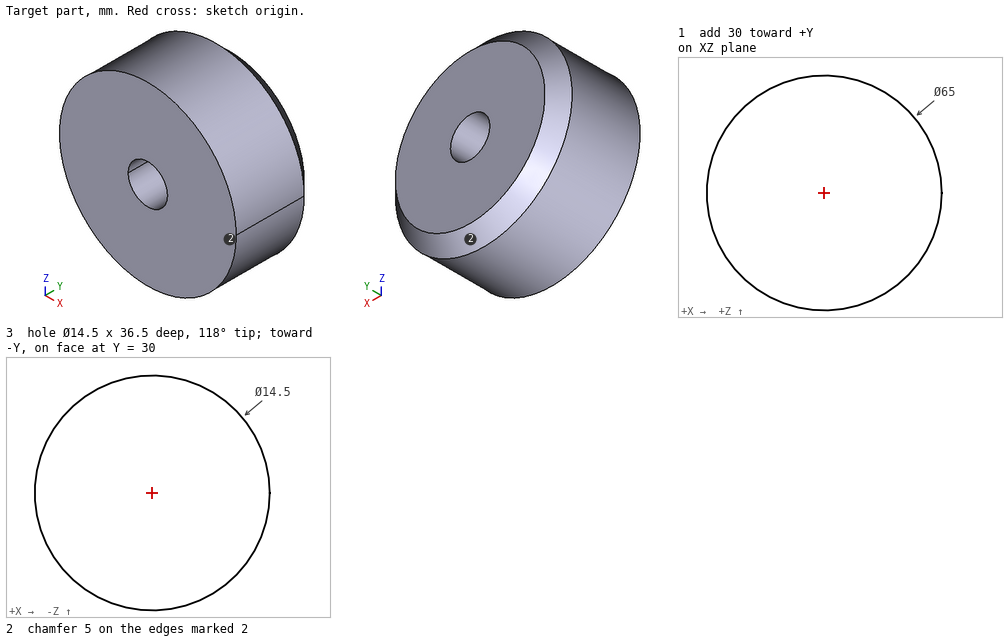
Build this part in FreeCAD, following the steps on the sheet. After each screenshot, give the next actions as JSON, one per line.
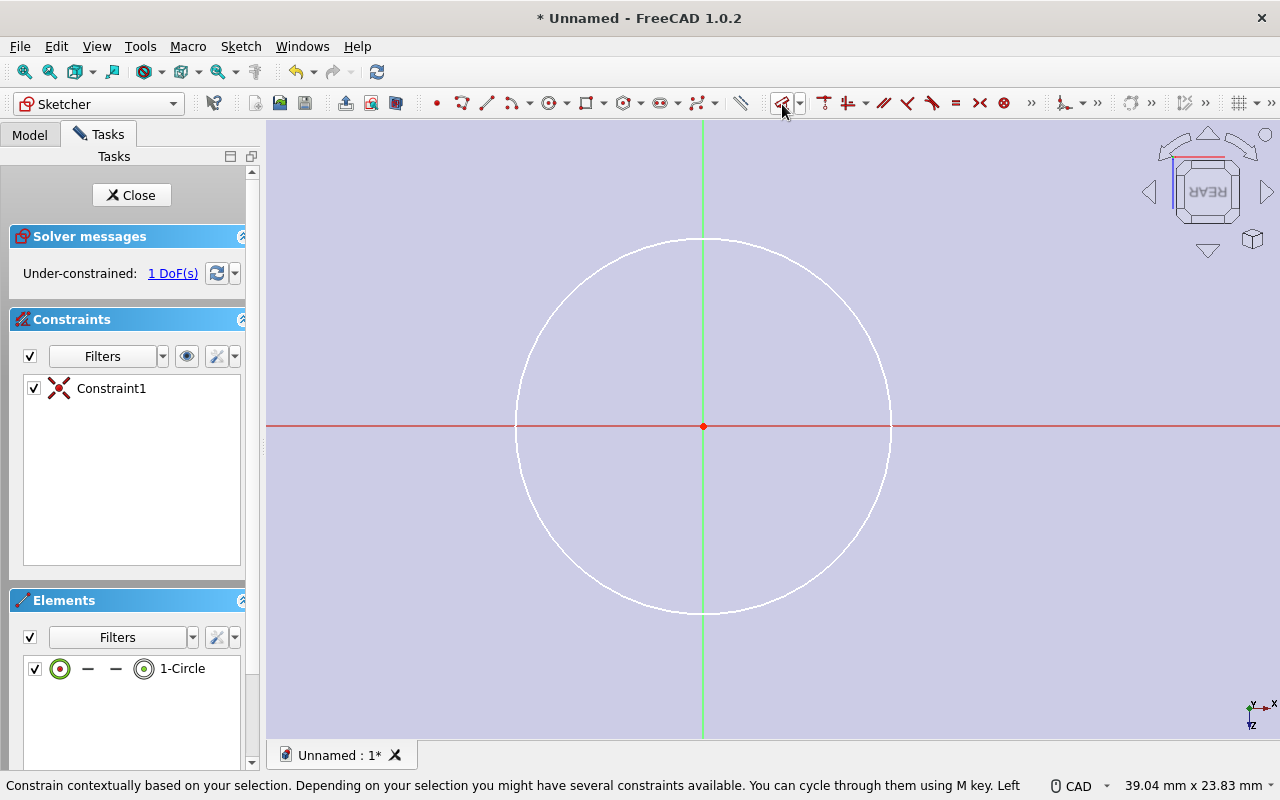
{"action": "left_click", "coordinate": [836, 293]}
{"action": "left_click", "coordinate": [859, 270]}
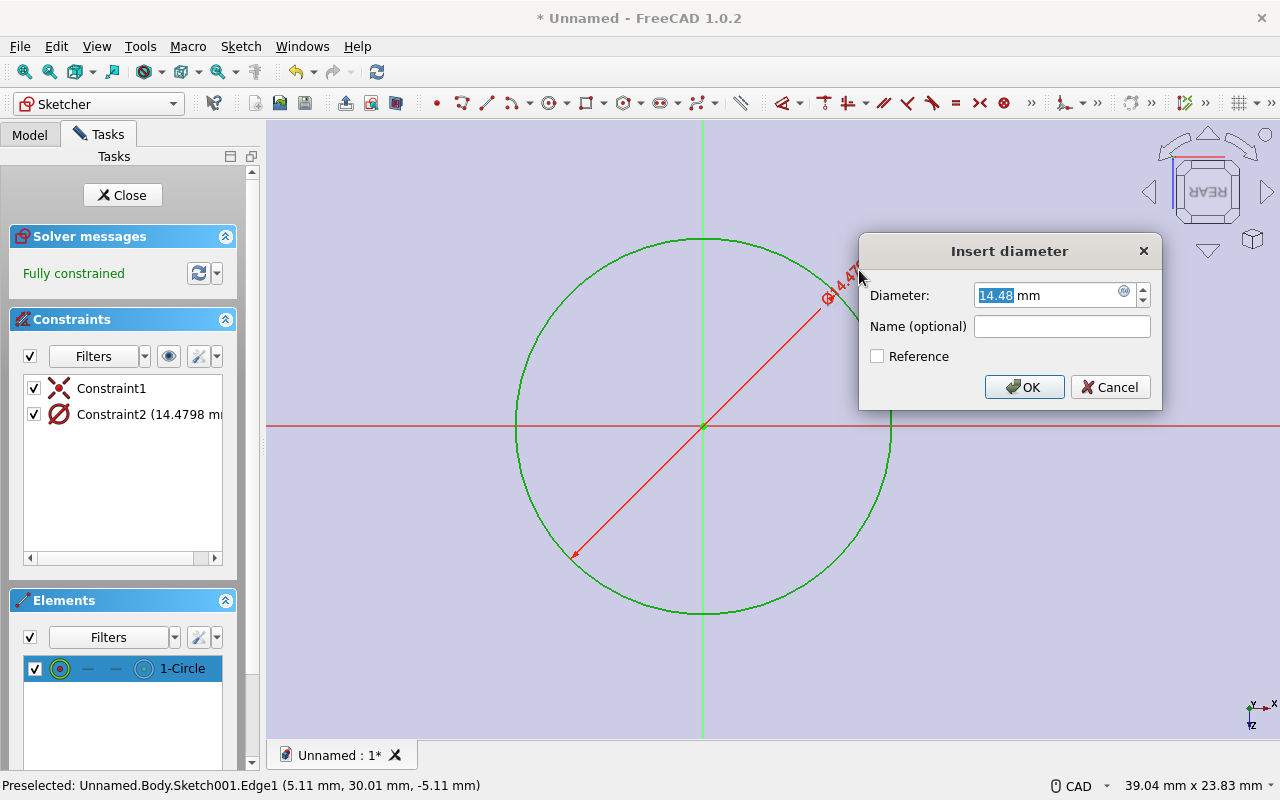
{"action": "type", "text": "14.5"}
{"action": "key", "text": "Return"}
{"action": "key", "text": "Escape"}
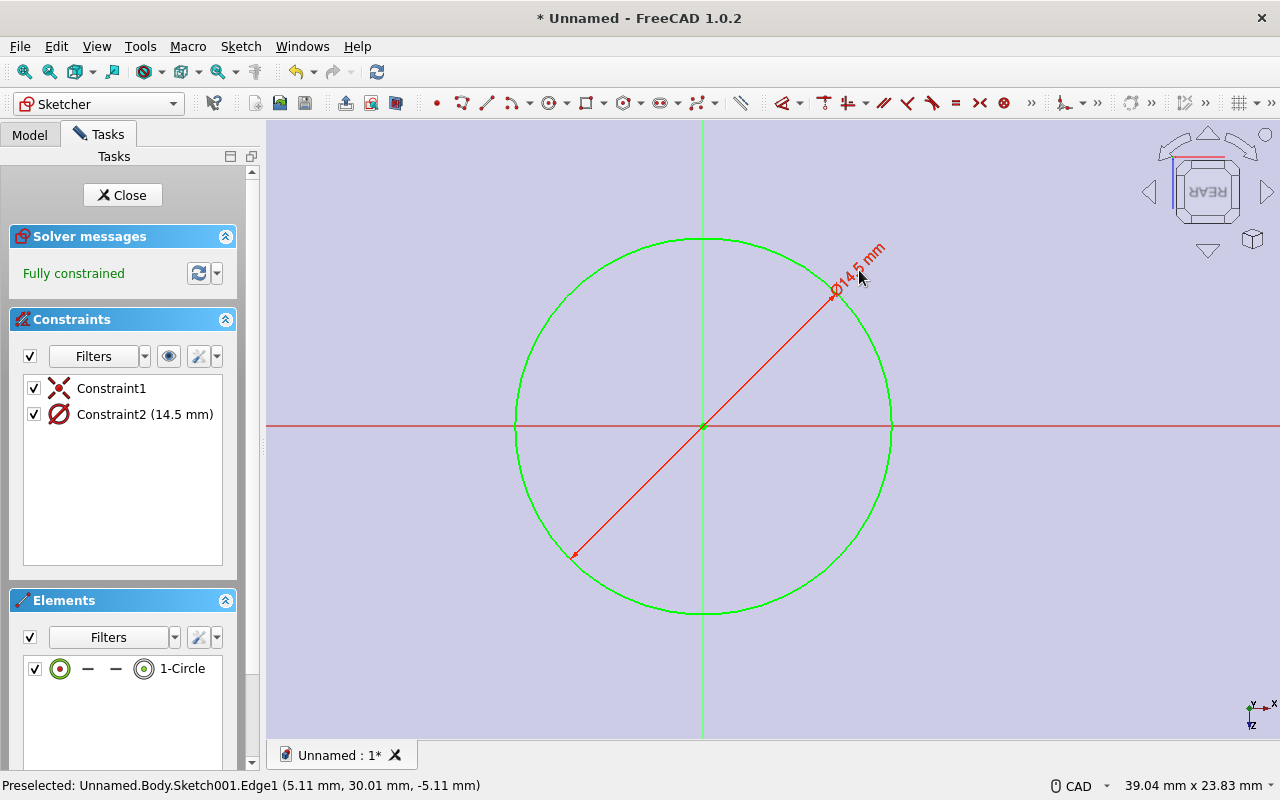
{"action": "left_click", "coordinate": [123, 195]}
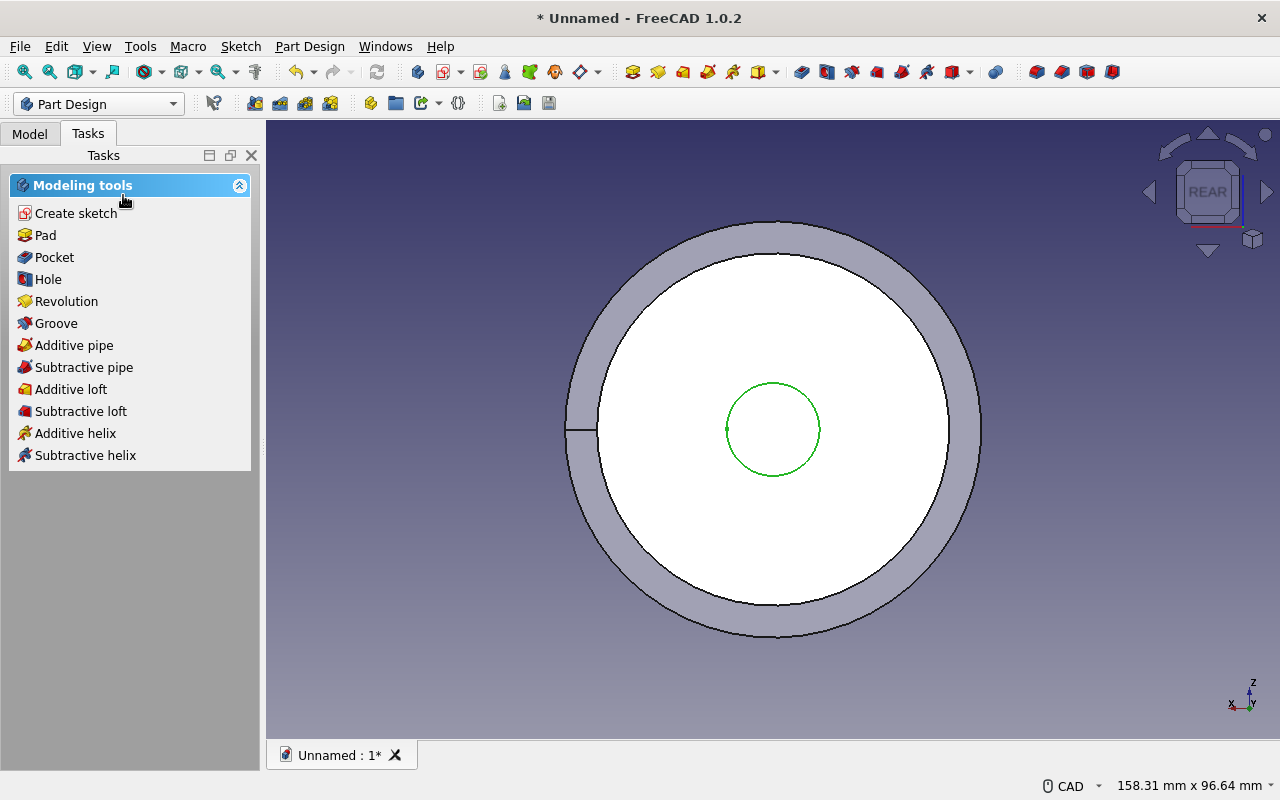
{"action": "left_click", "coordinate": [827, 72]}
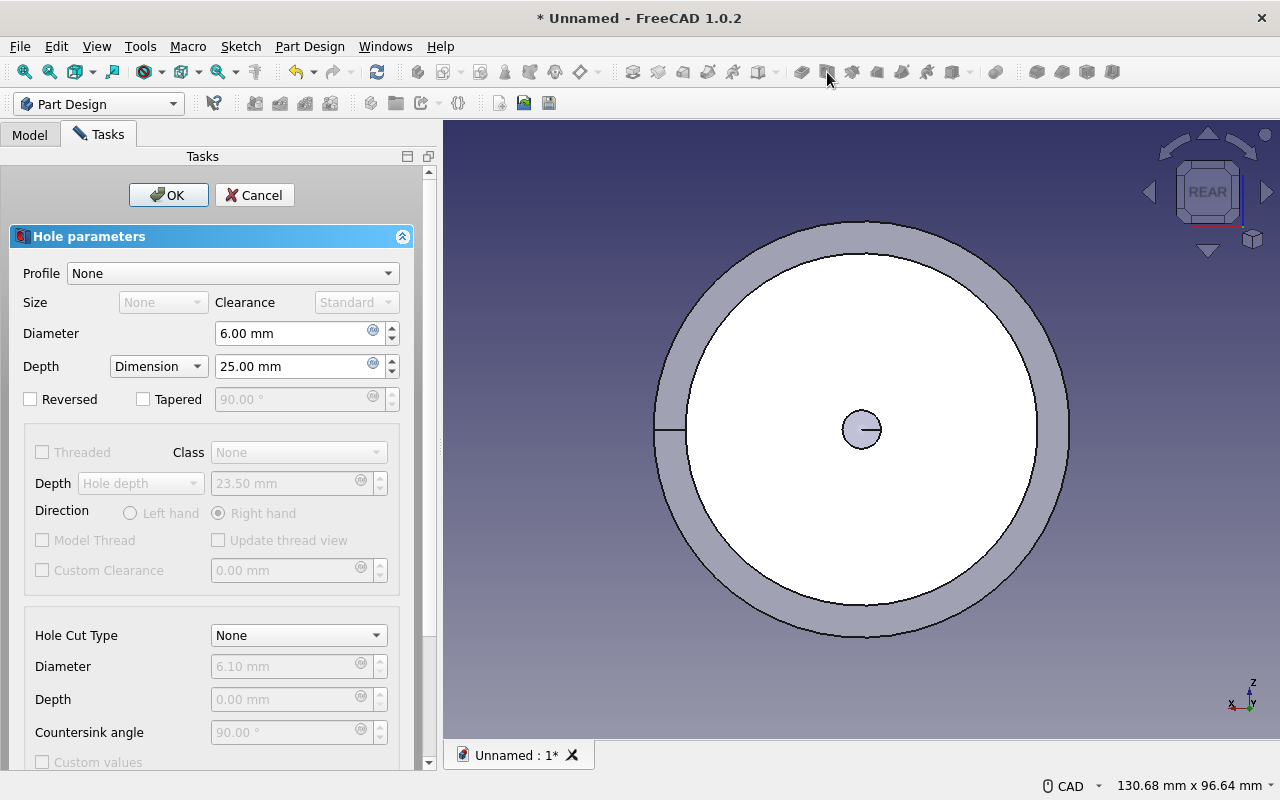
{"action": "triple_click", "coordinate": [300, 334]}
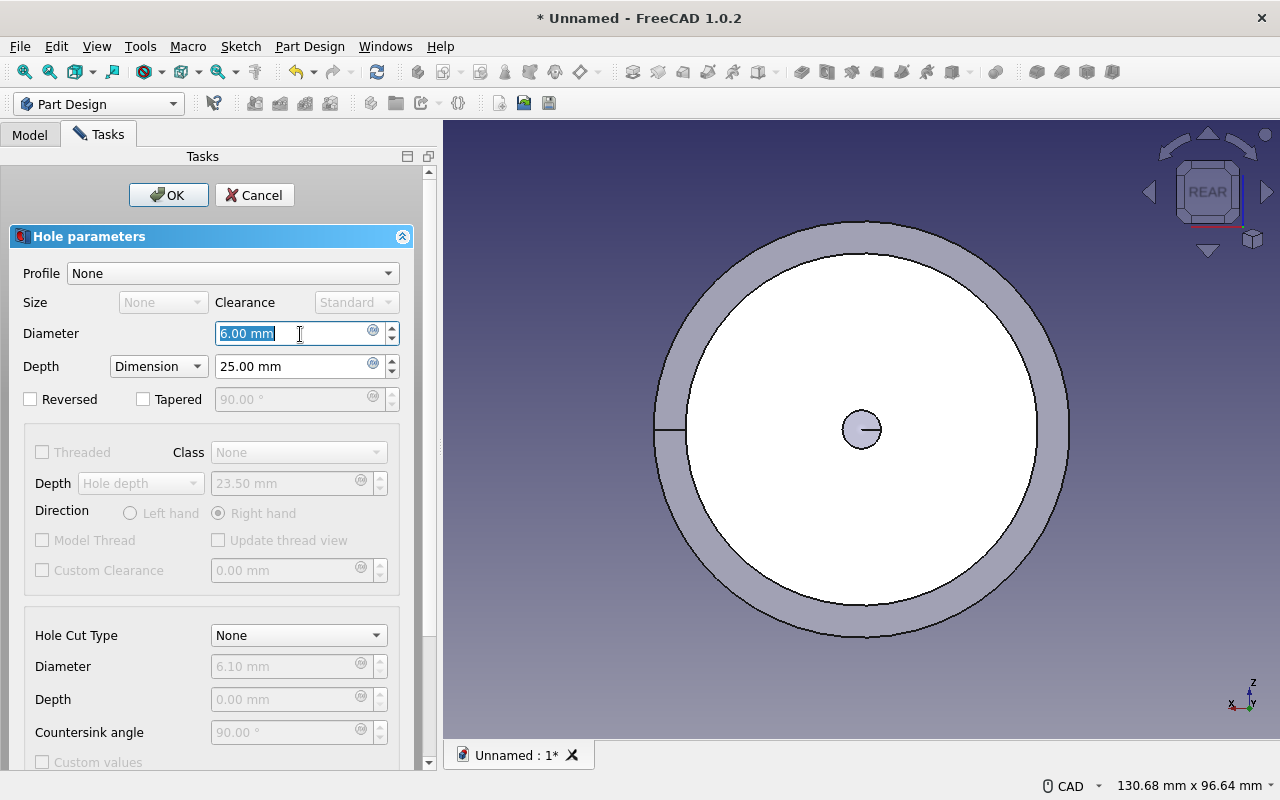
{"action": "type", "text": "14.5"}
{"action": "key", "text": "Tab"}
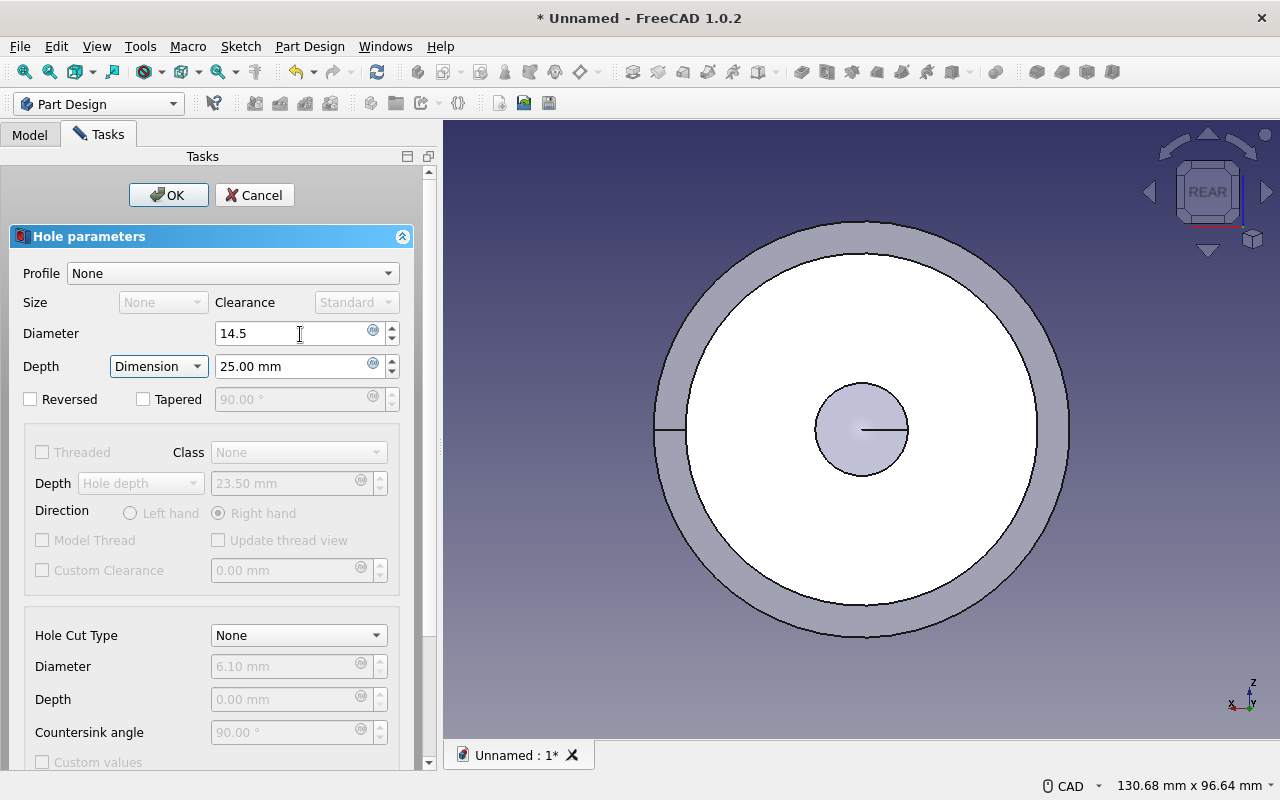
{"action": "triple_click", "coordinate": [300, 366]}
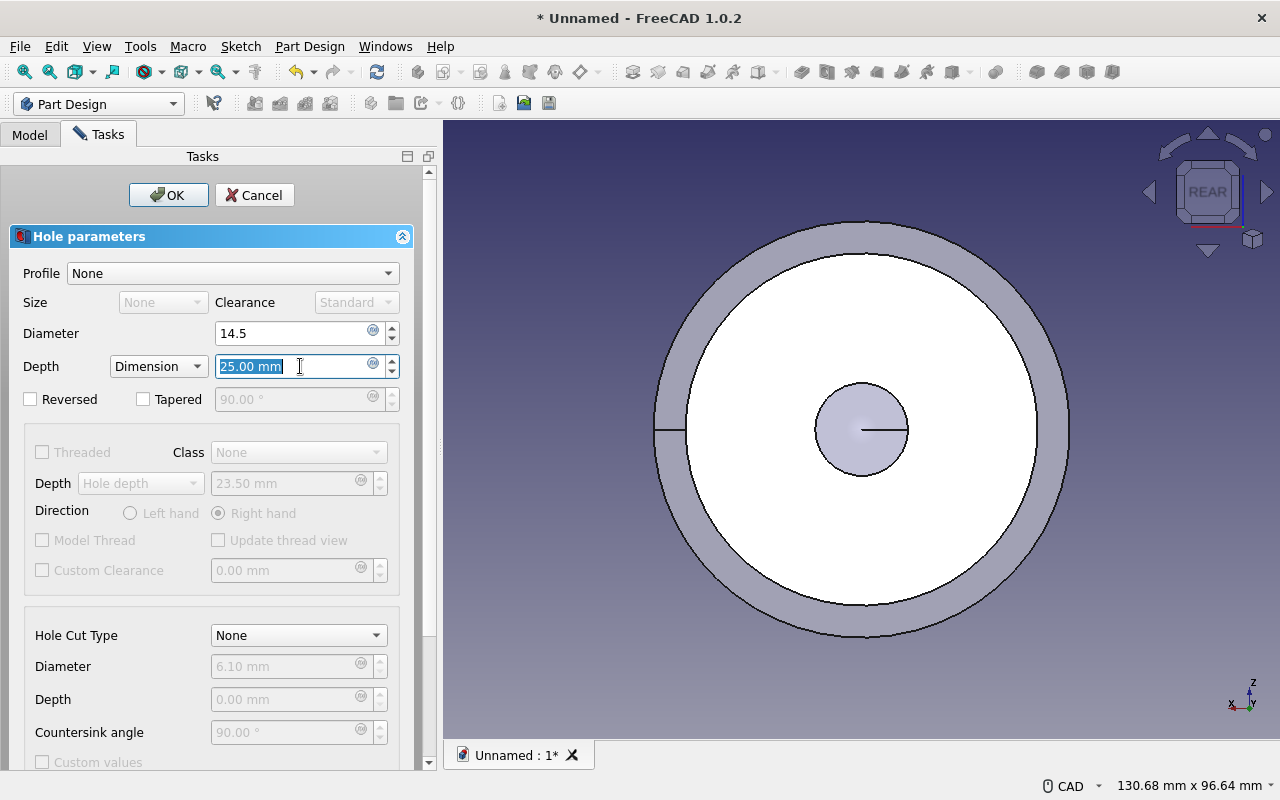
{"action": "type", "text": "36.5"}
{"action": "key", "text": "Tab"}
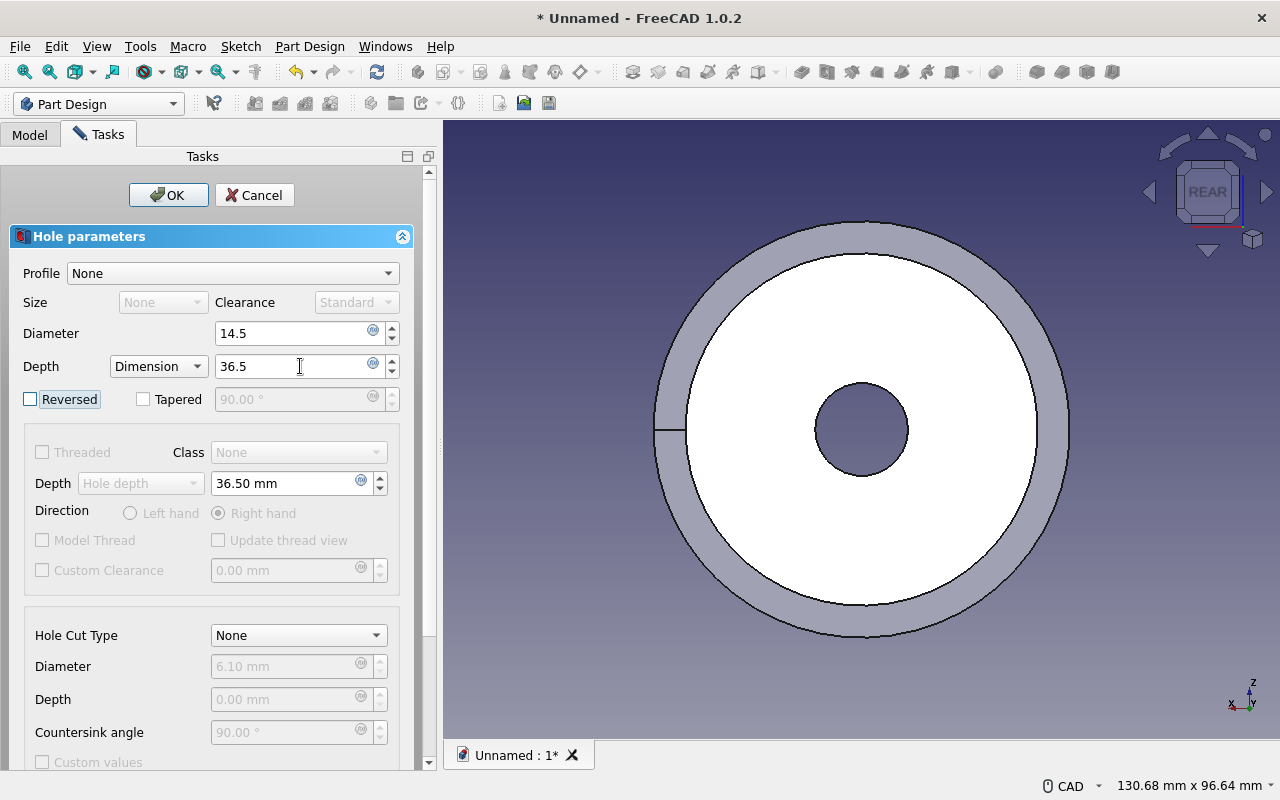
{"action": "left_click", "coordinate": [169, 195]}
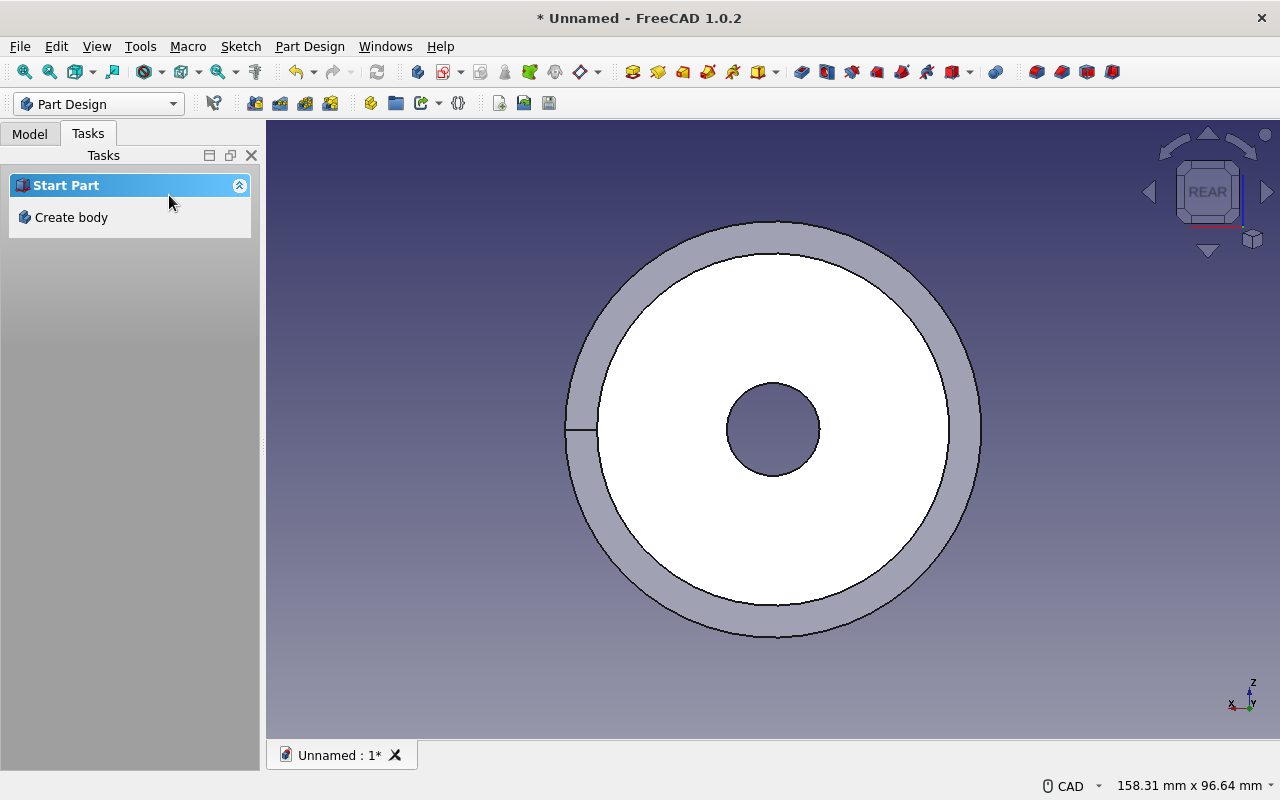
{"action": "key", "text": "0"}